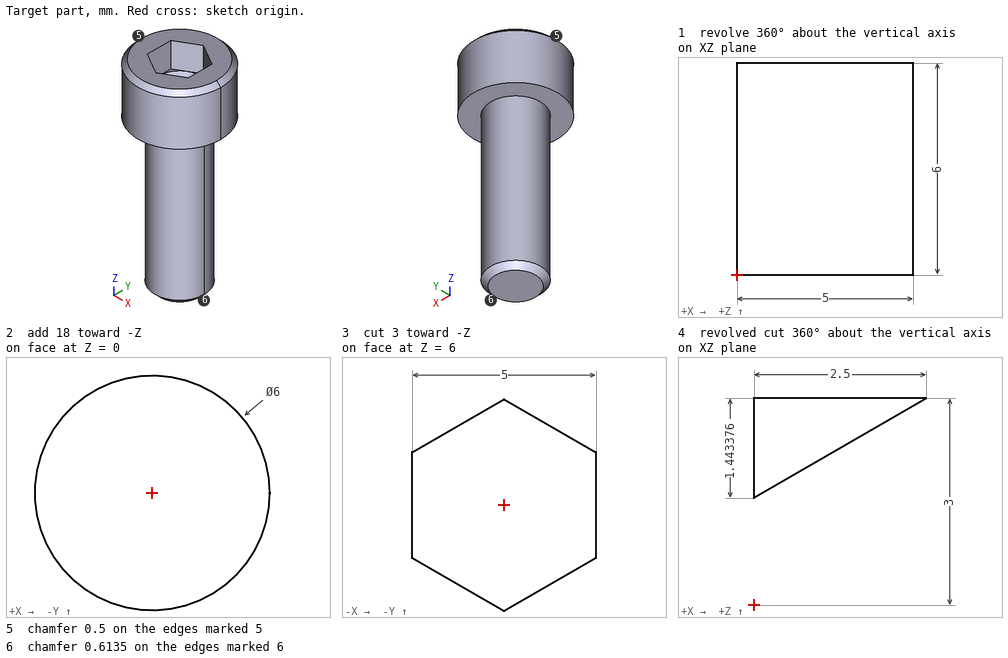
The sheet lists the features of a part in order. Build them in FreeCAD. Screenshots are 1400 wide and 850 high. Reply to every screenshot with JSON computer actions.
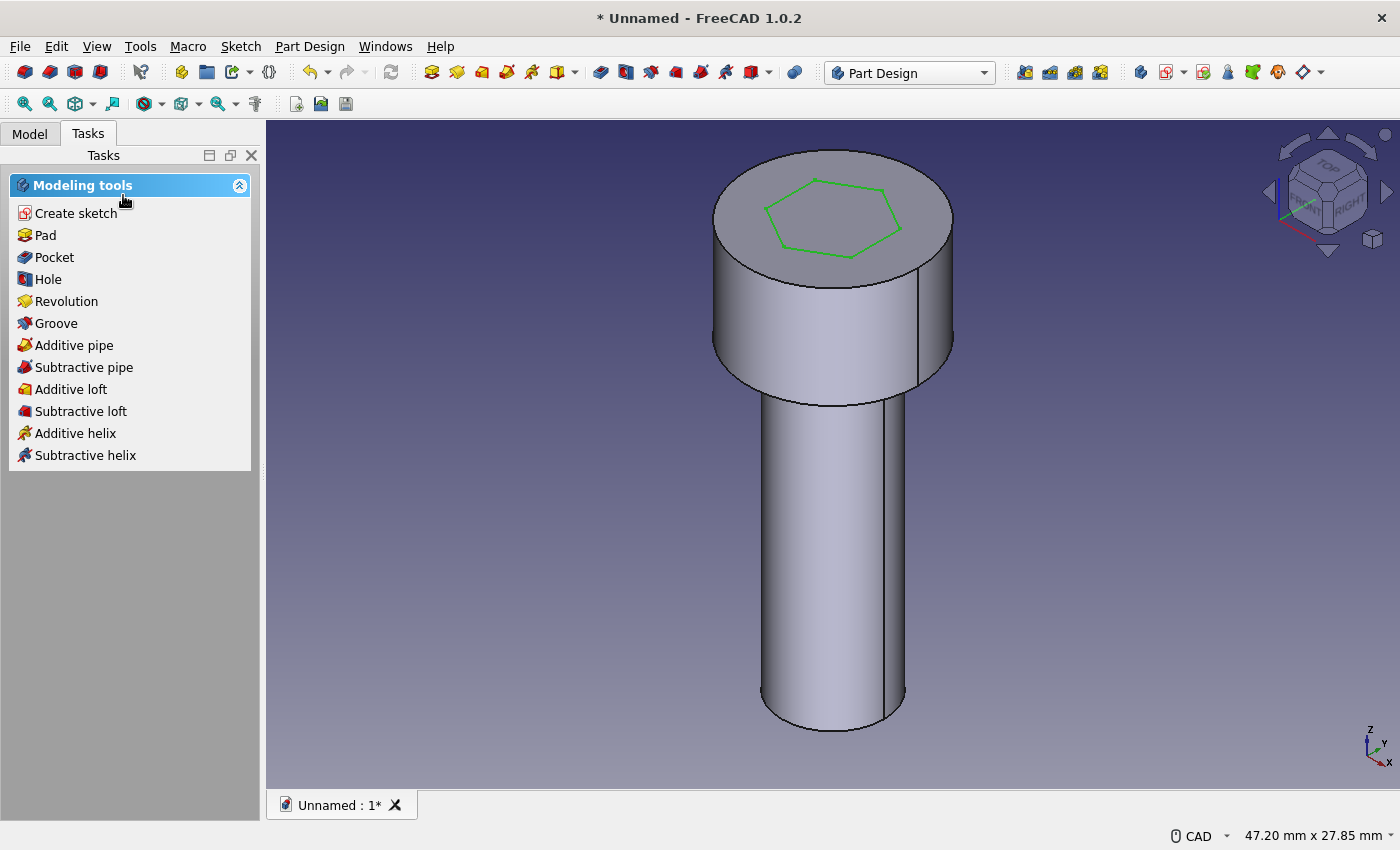
{"action": "left_click", "coordinate": [601, 72]}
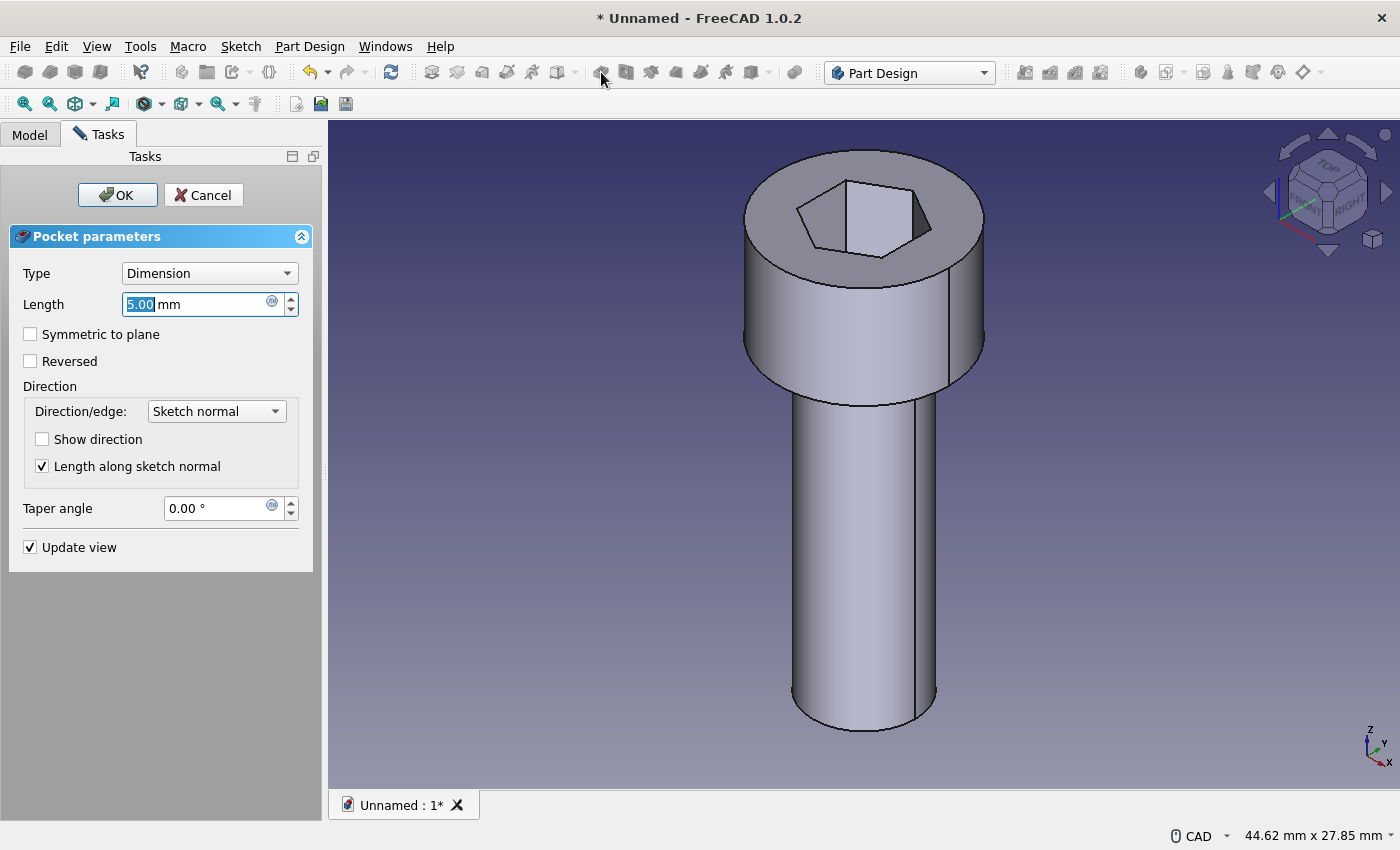
{"action": "type", "text": "3"}
{"action": "key", "text": "Tab"}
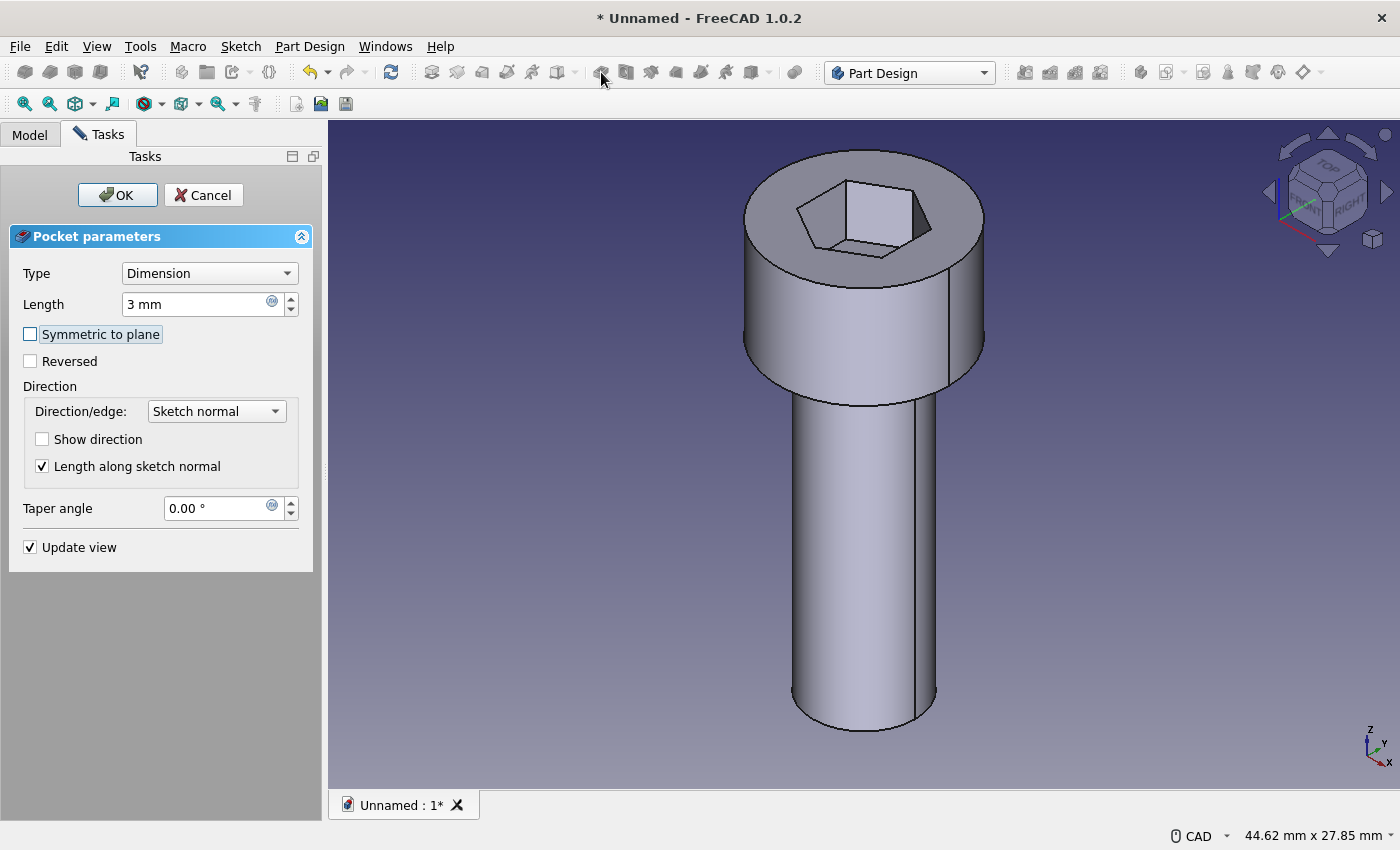
{"action": "left_click", "coordinate": [118, 195]}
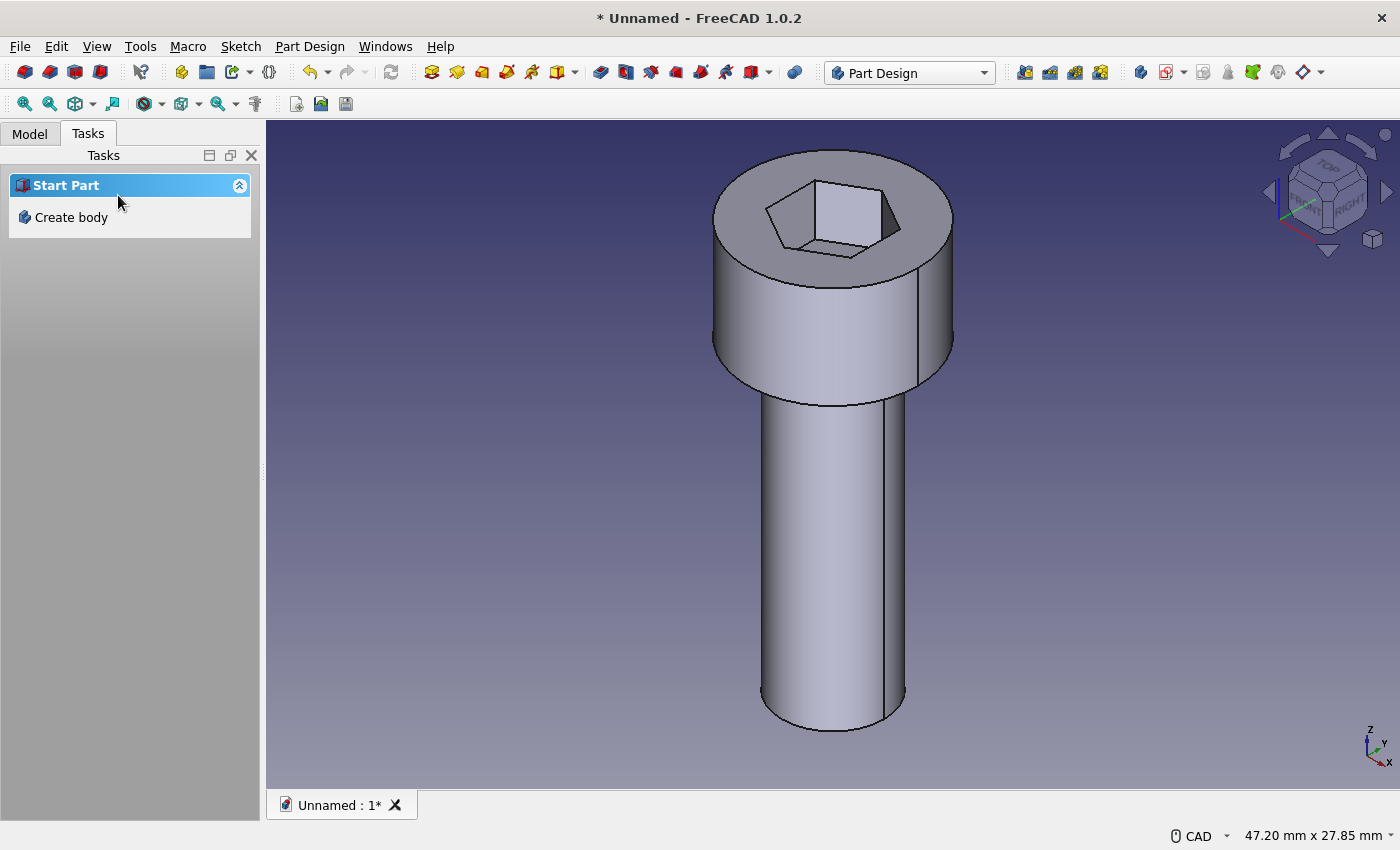
{"action": "left_click", "coordinate": [1166, 72]}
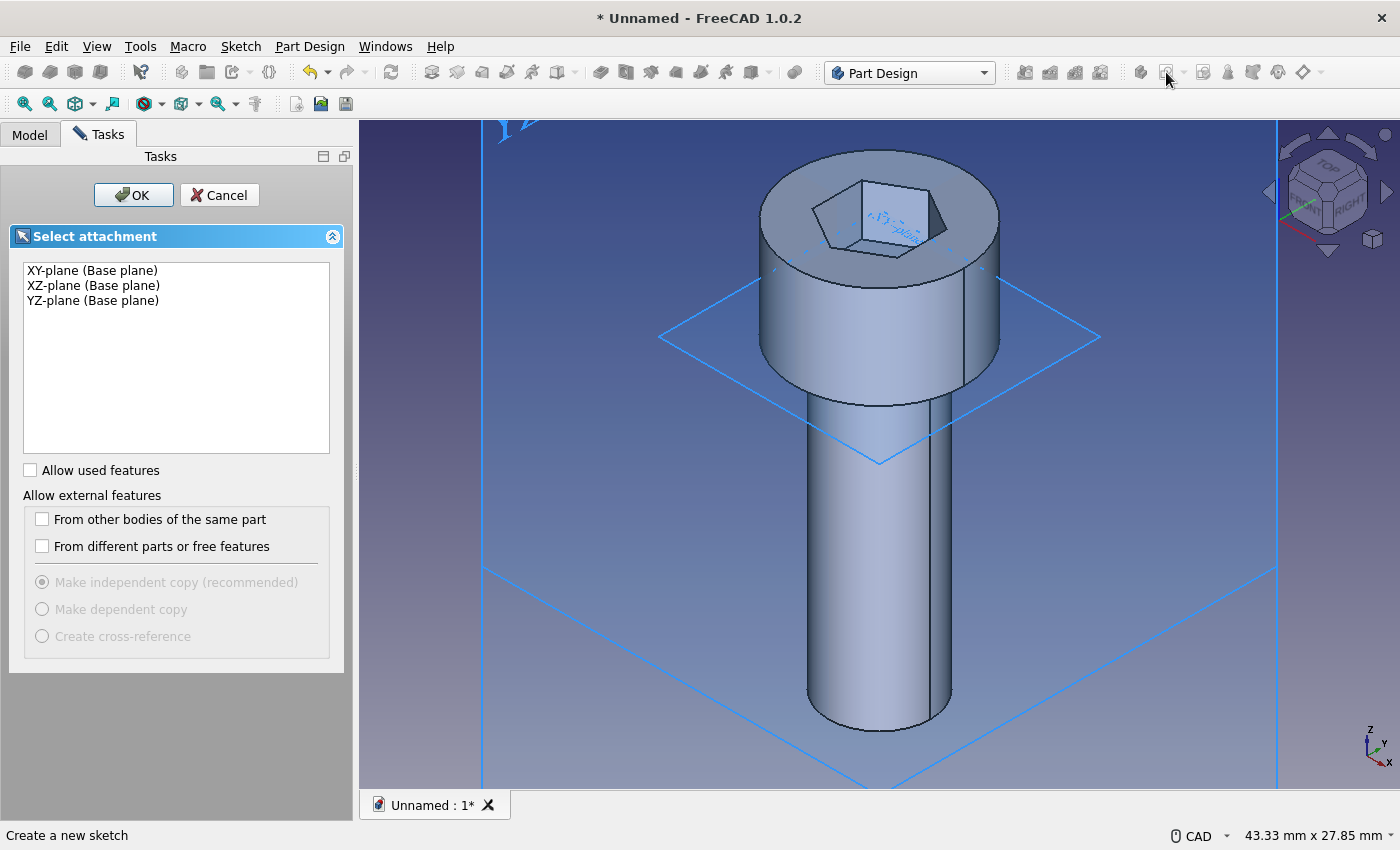
{"action": "left_click", "coordinate": [84, 286]}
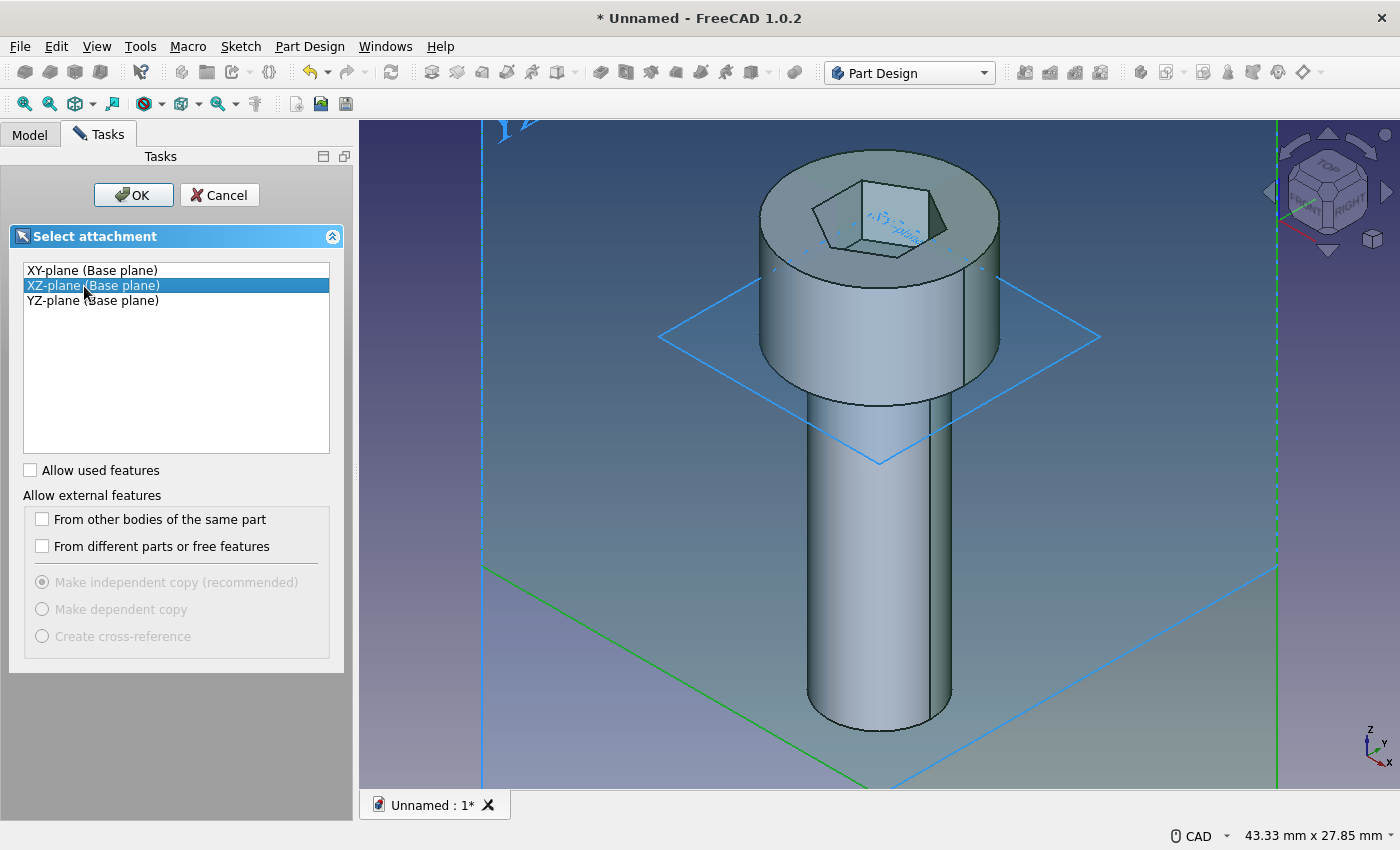
{"action": "left_click", "coordinate": [134, 195]}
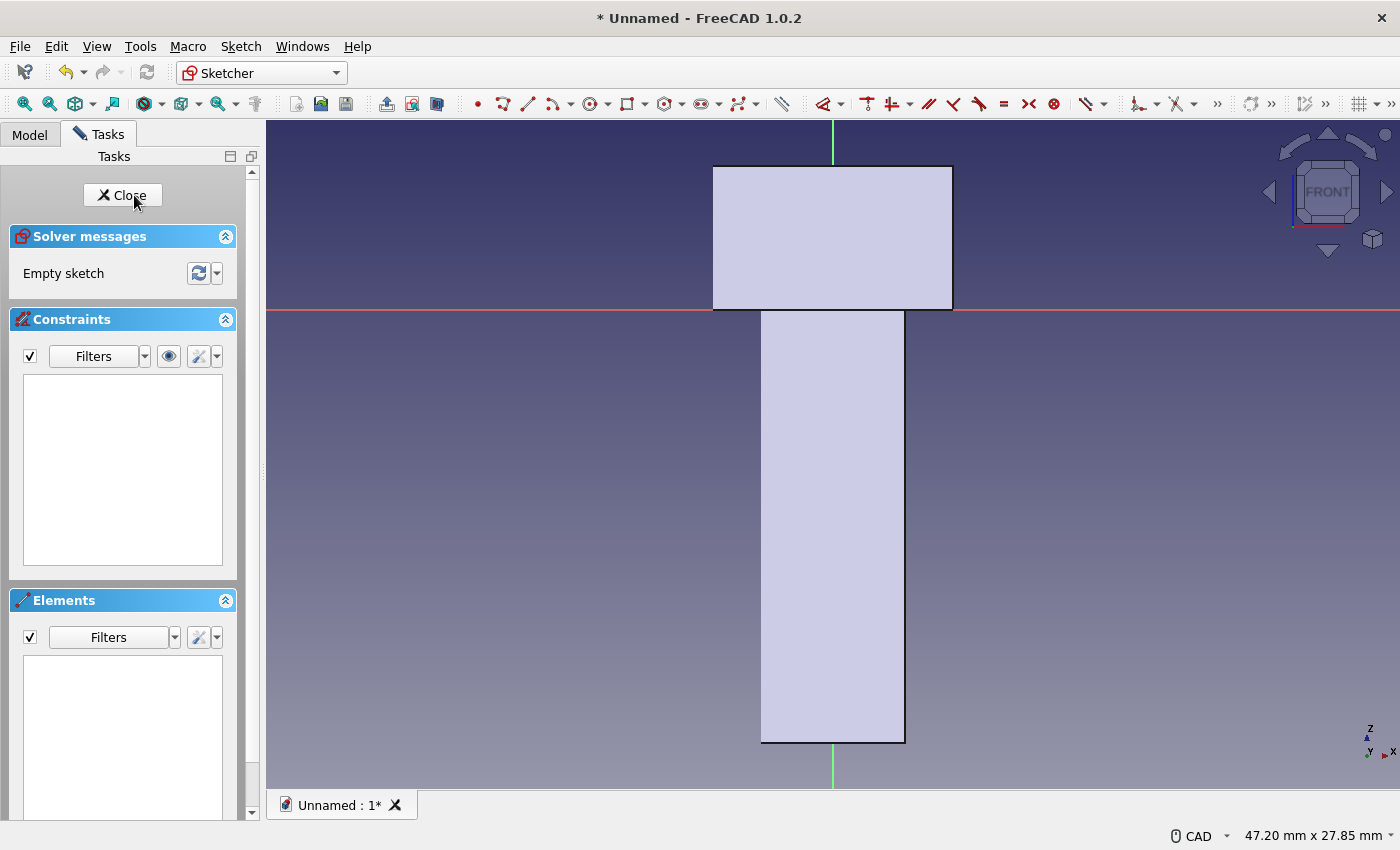
{"action": "left_click", "coordinate": [437, 104]}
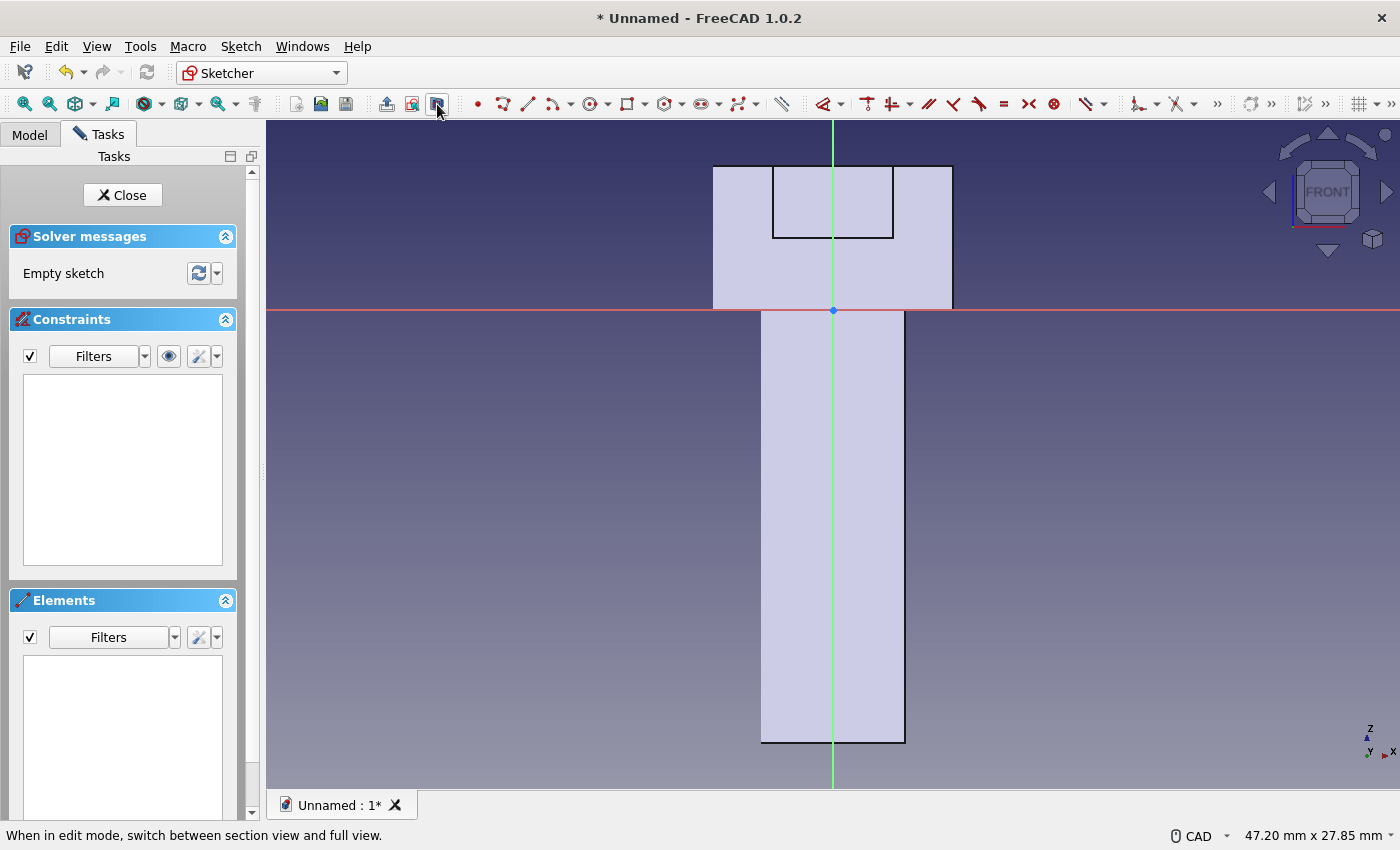
{"action": "scroll", "coordinate": [883, 239], "scroll_direction": "up", "scroll_amount": 9}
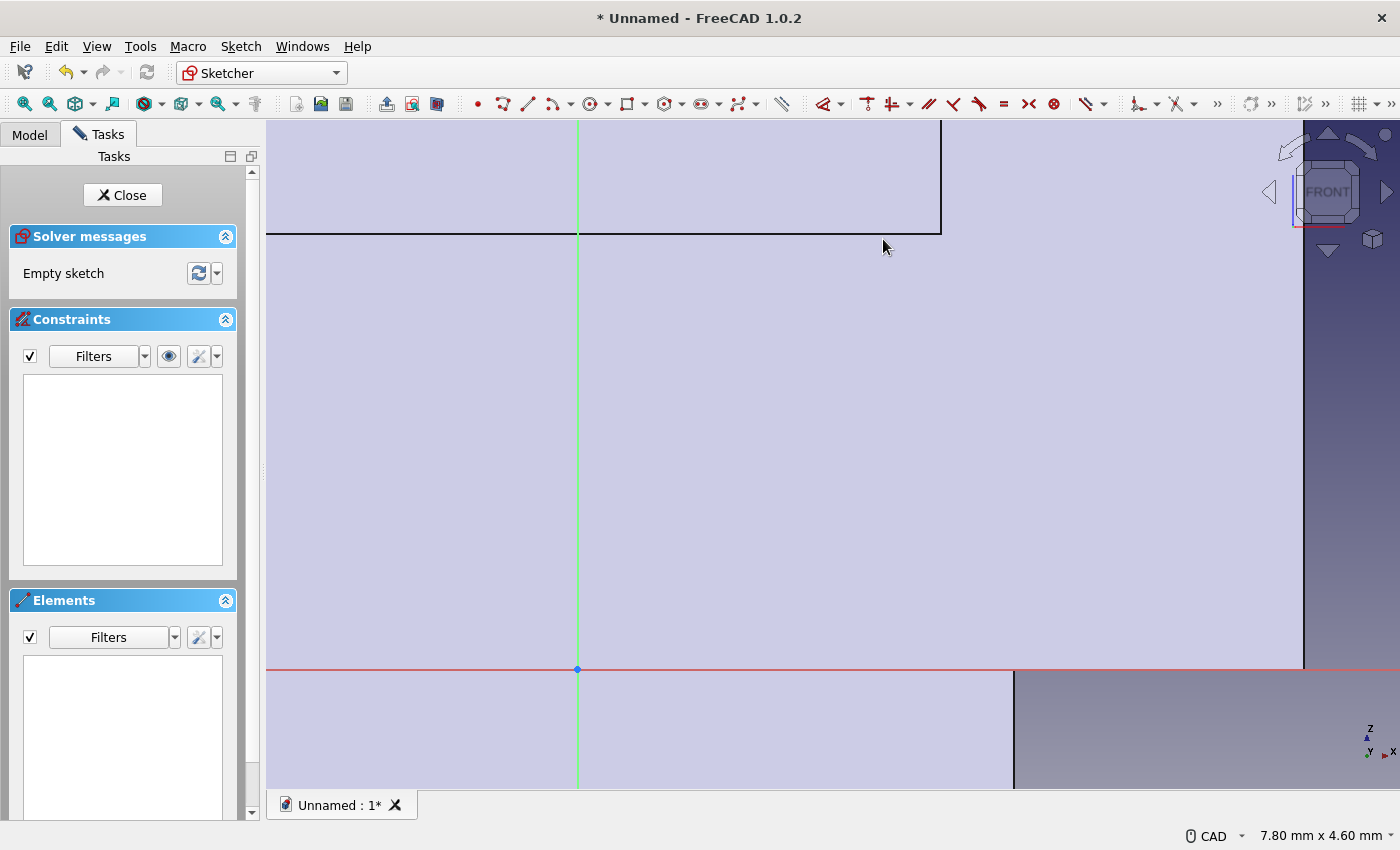
{"action": "left_click", "coordinate": [503, 104]}